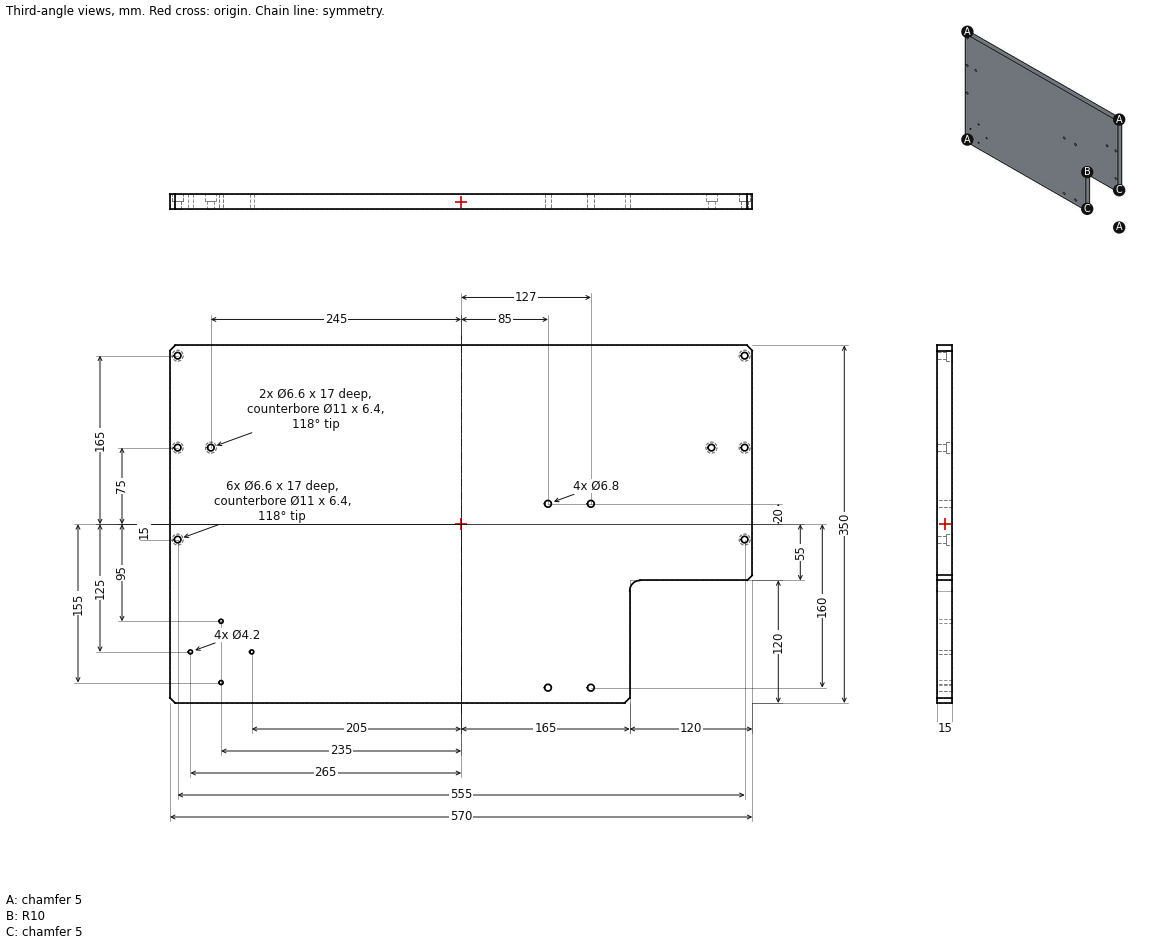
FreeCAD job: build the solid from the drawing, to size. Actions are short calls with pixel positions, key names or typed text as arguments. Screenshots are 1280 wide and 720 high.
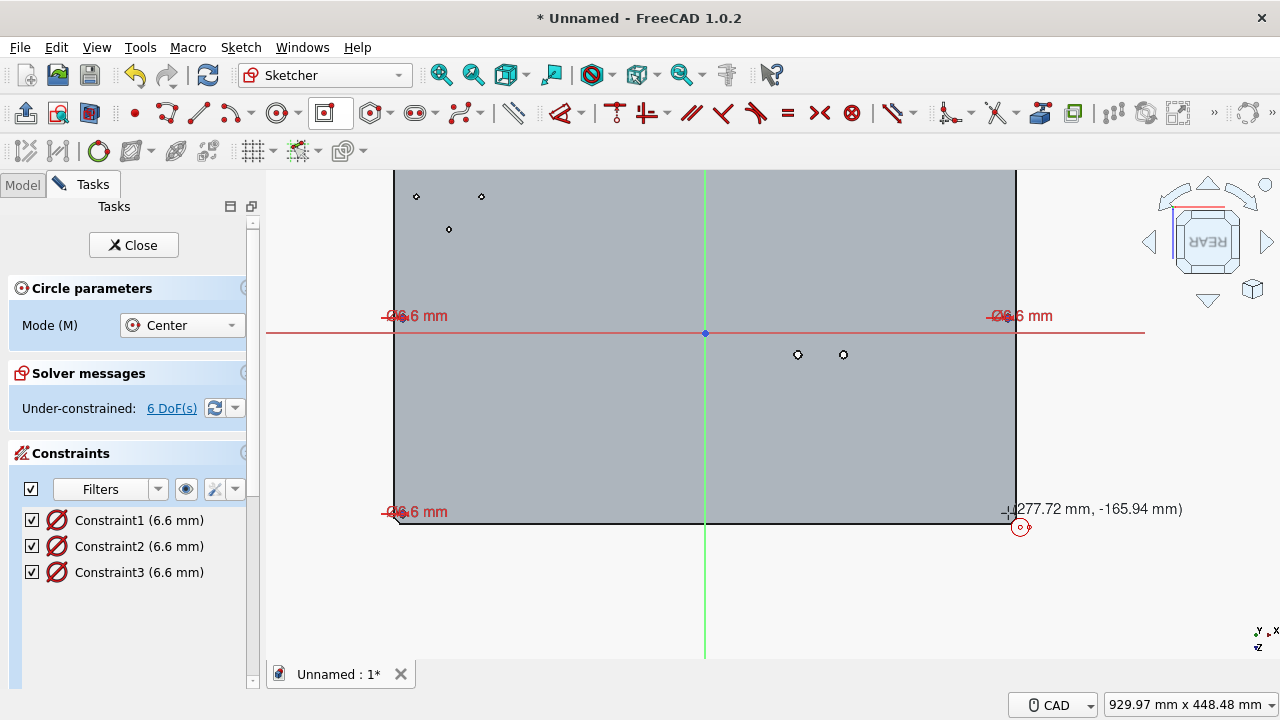
click(1008, 513)
move(1010, 510)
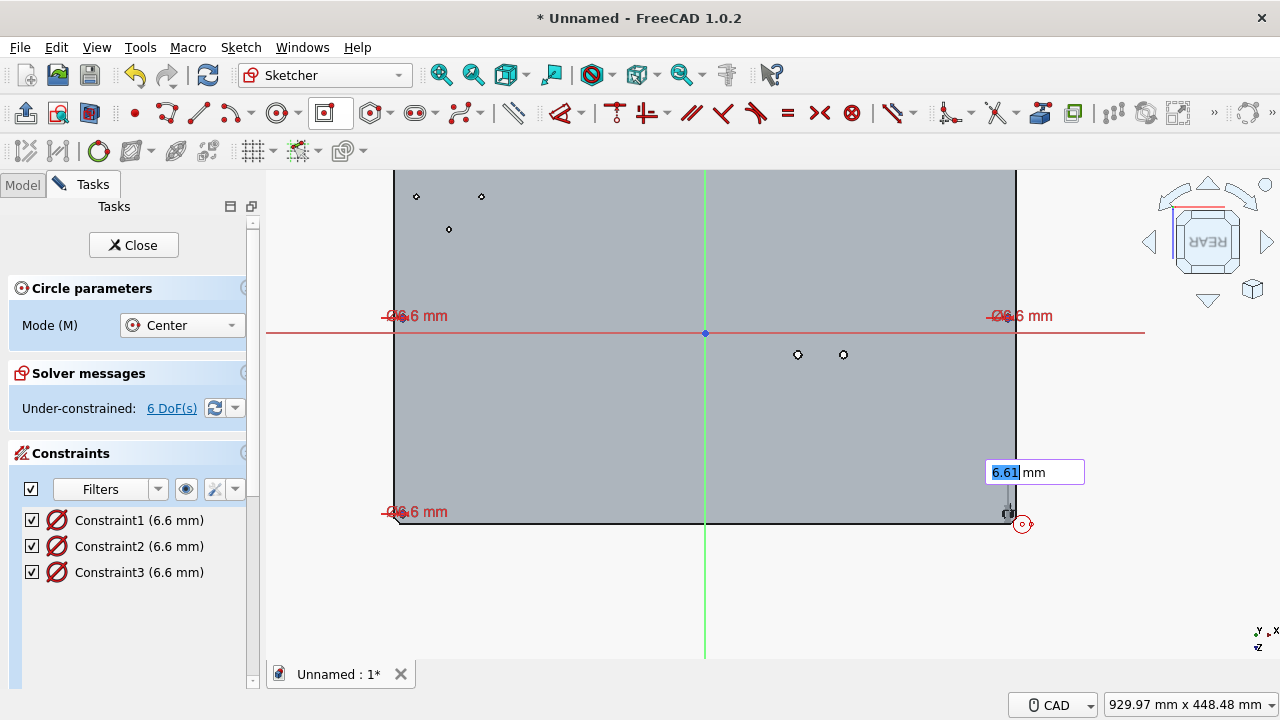
text(6.6)
key(Return)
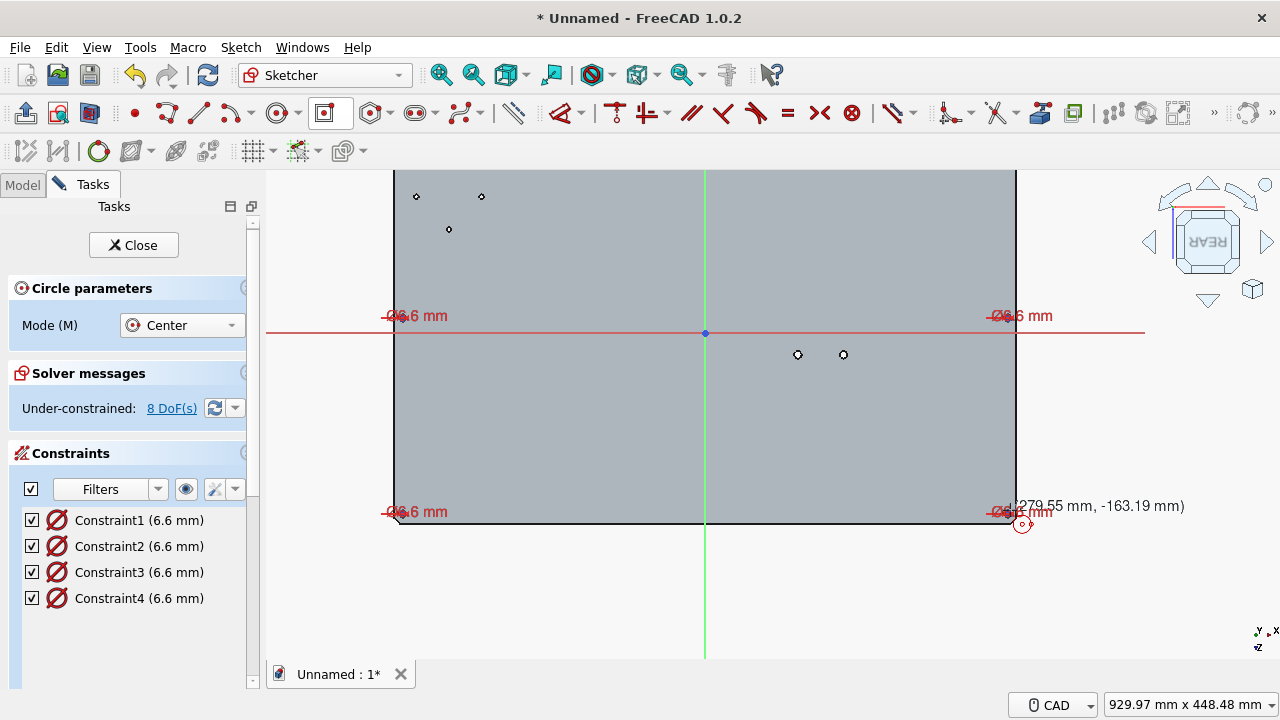
scroll(403, 415, up, 10)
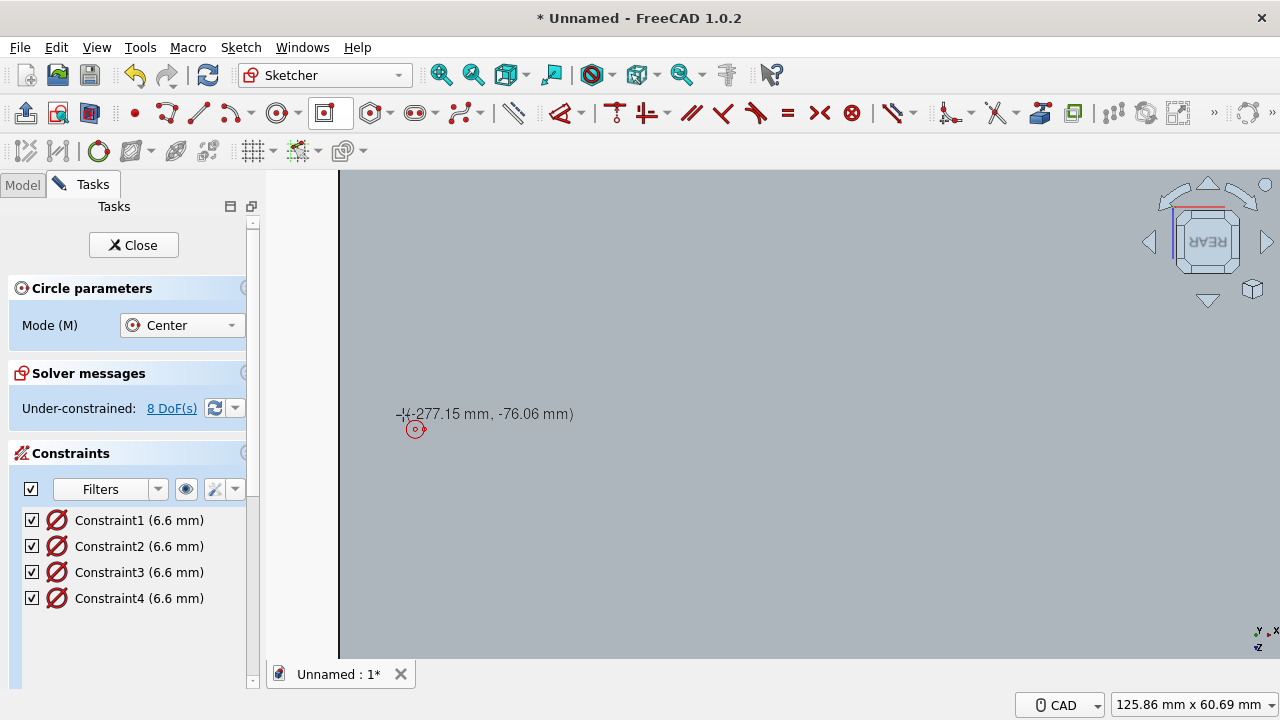
scroll(402, 415, down, 10)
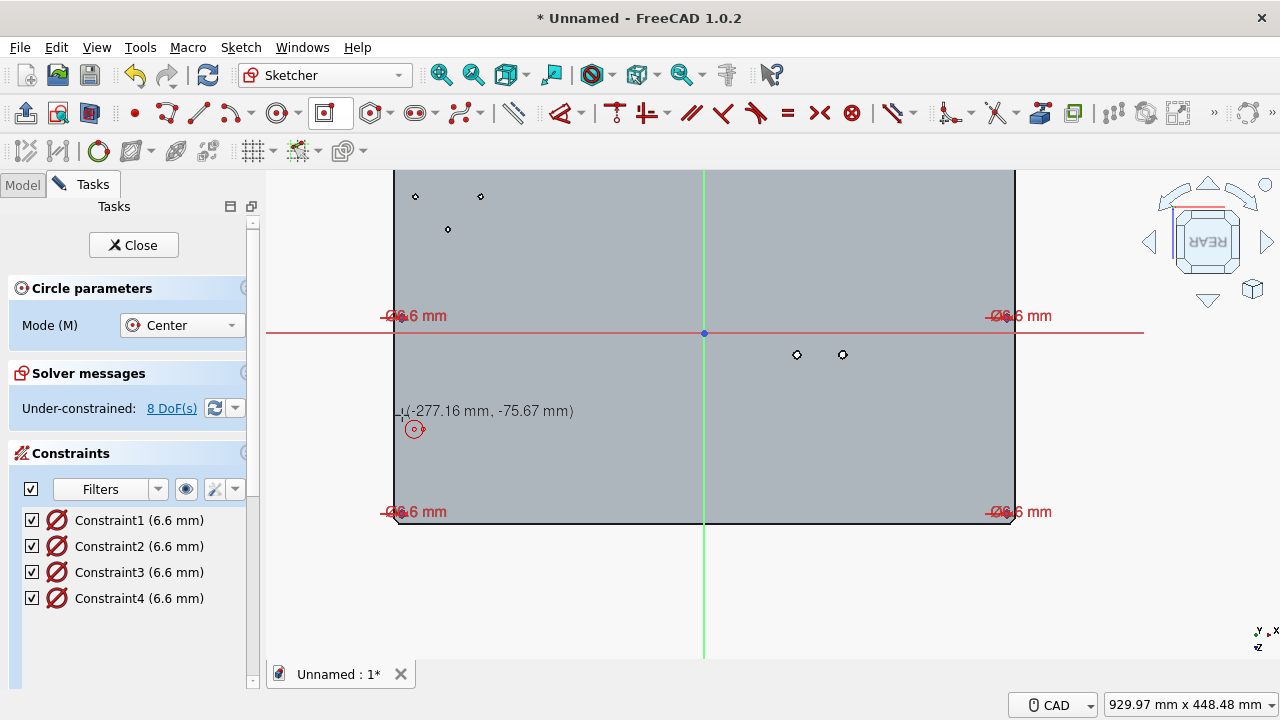
click(402, 415)
move(404, 412)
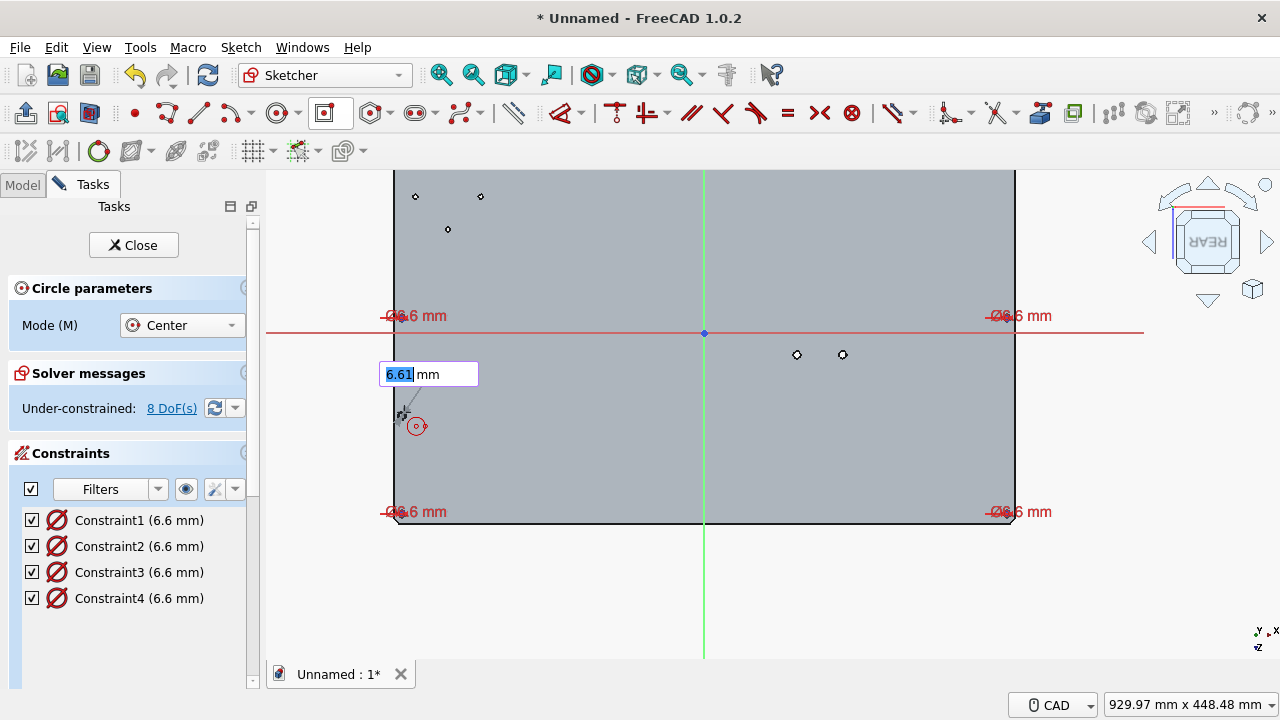
text(6.6)
key(Return)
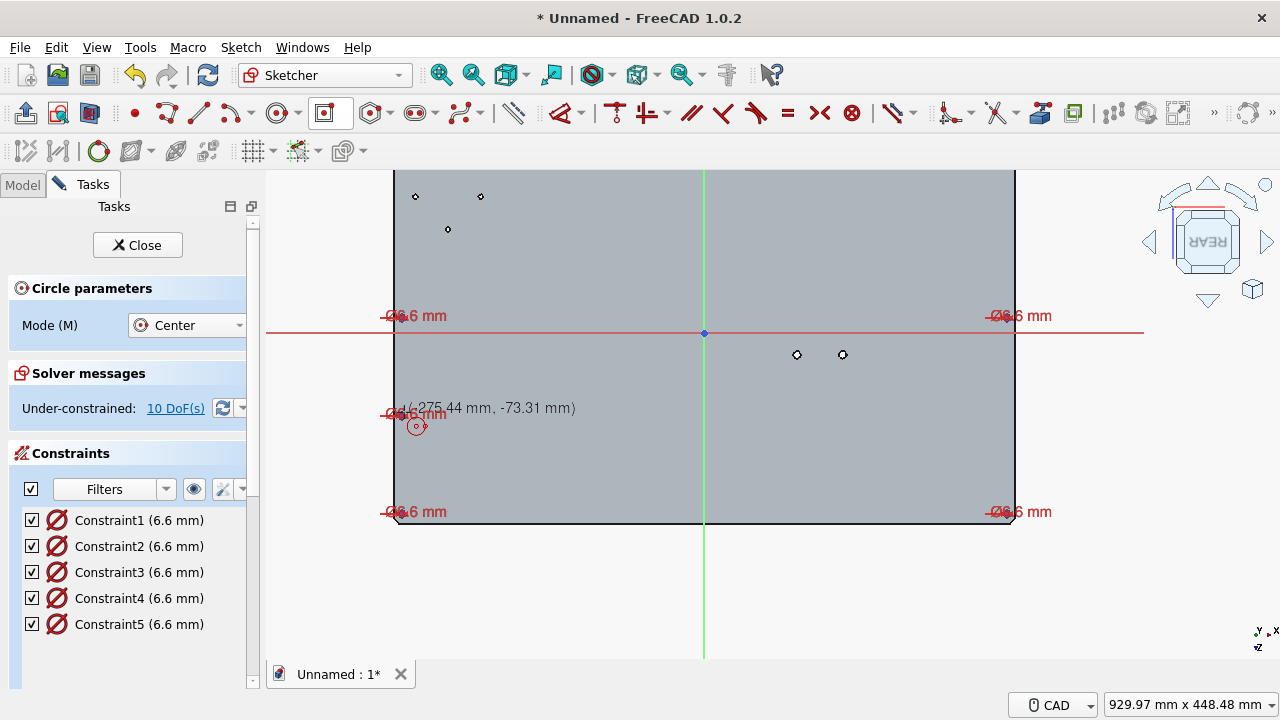
scroll(1007, 415, up, 10)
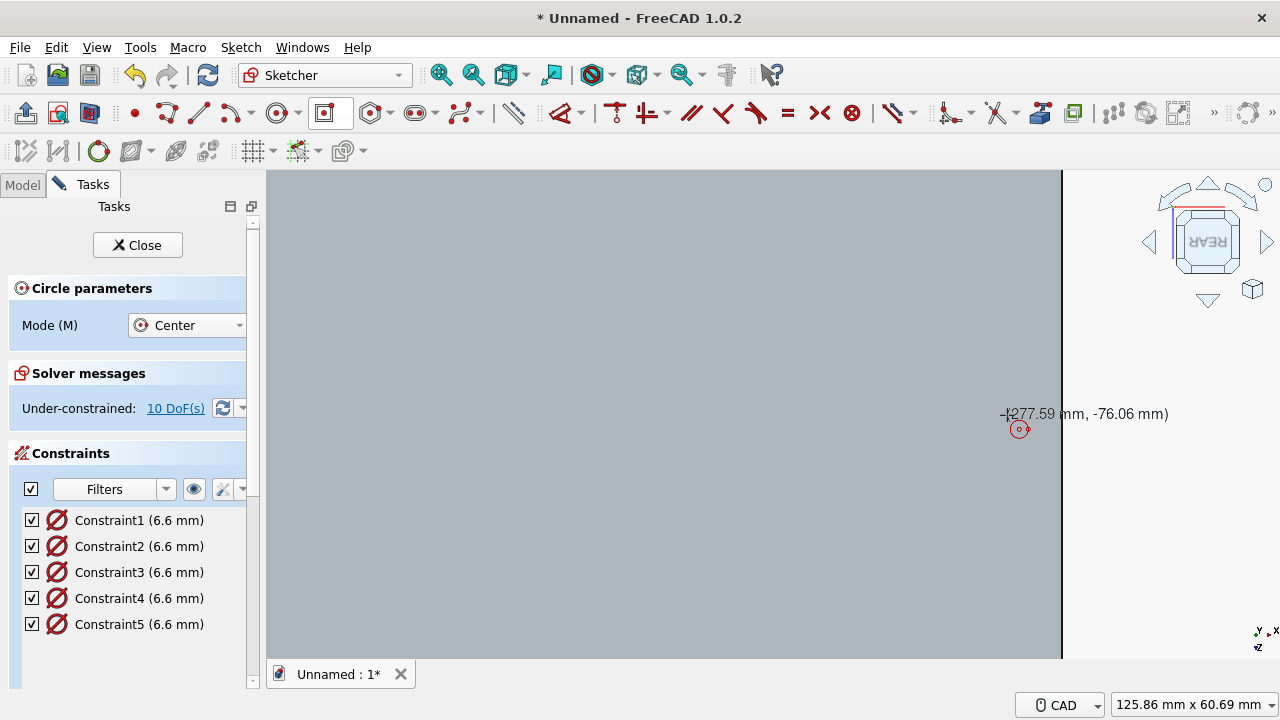
scroll(1008, 415, down, 10)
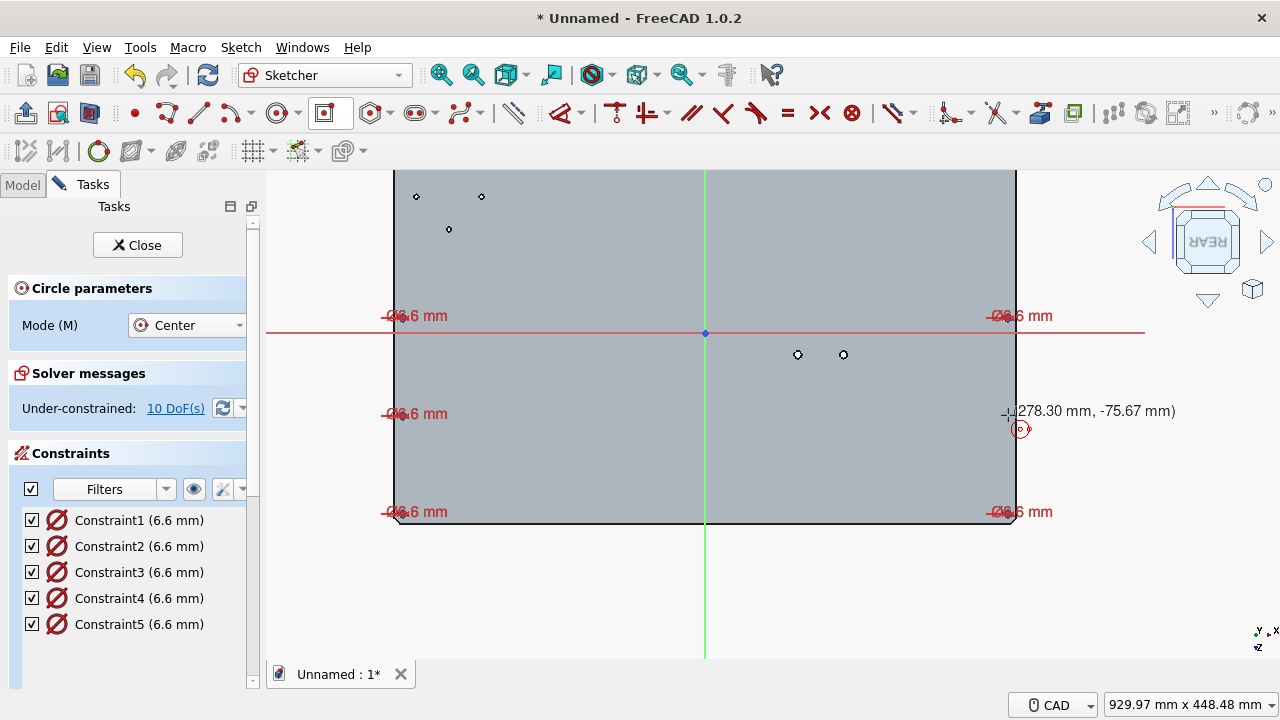
click(1008, 415)
move(1010, 412)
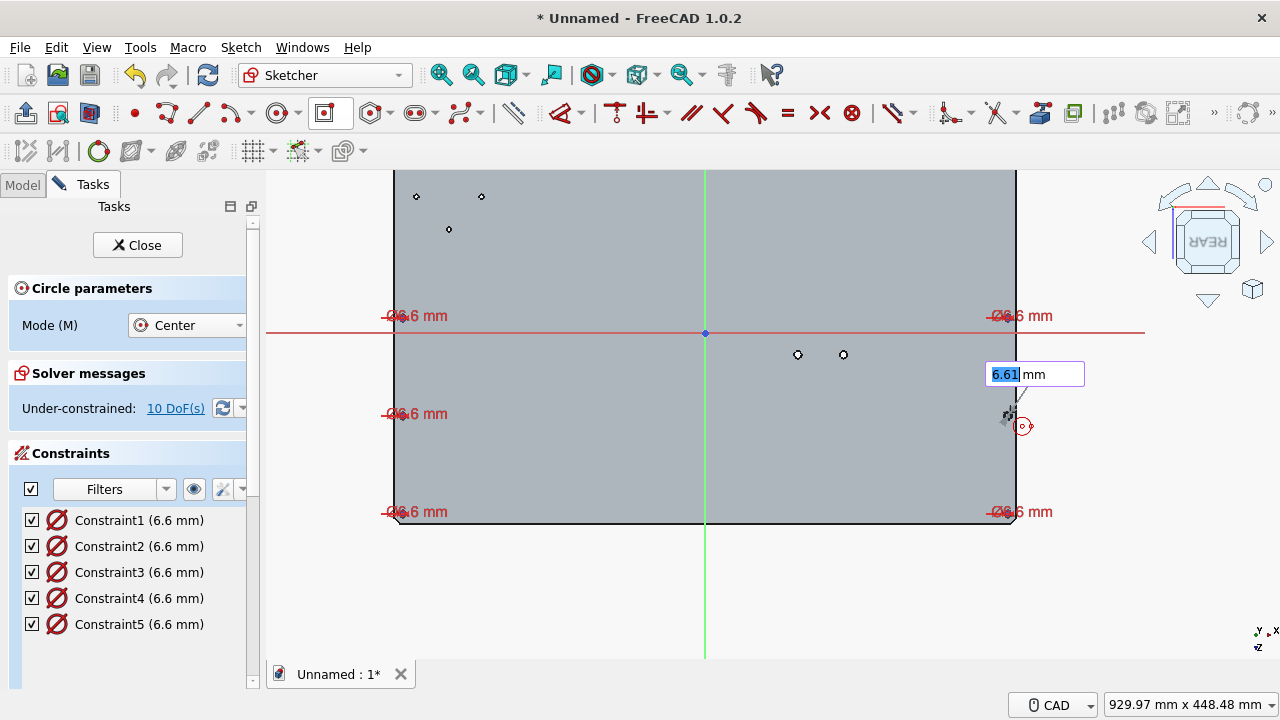
text(6.6)
key(Return)
key(Escape)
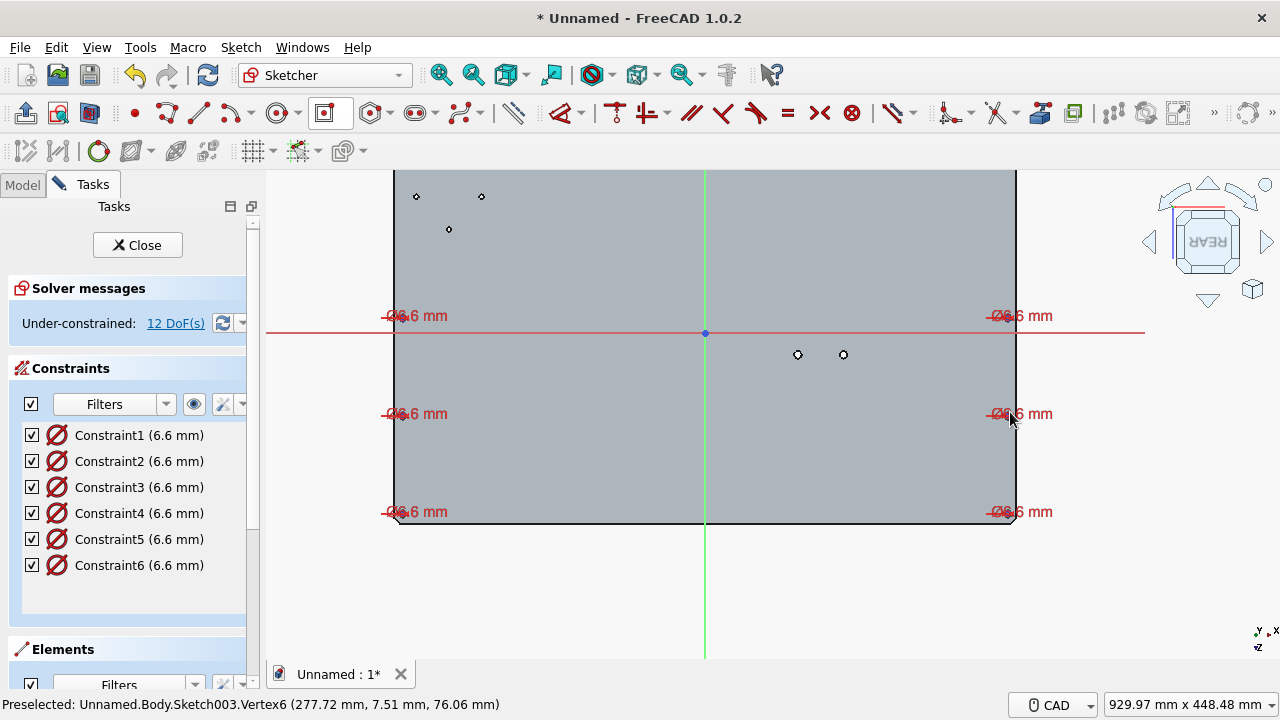
click(403, 318)